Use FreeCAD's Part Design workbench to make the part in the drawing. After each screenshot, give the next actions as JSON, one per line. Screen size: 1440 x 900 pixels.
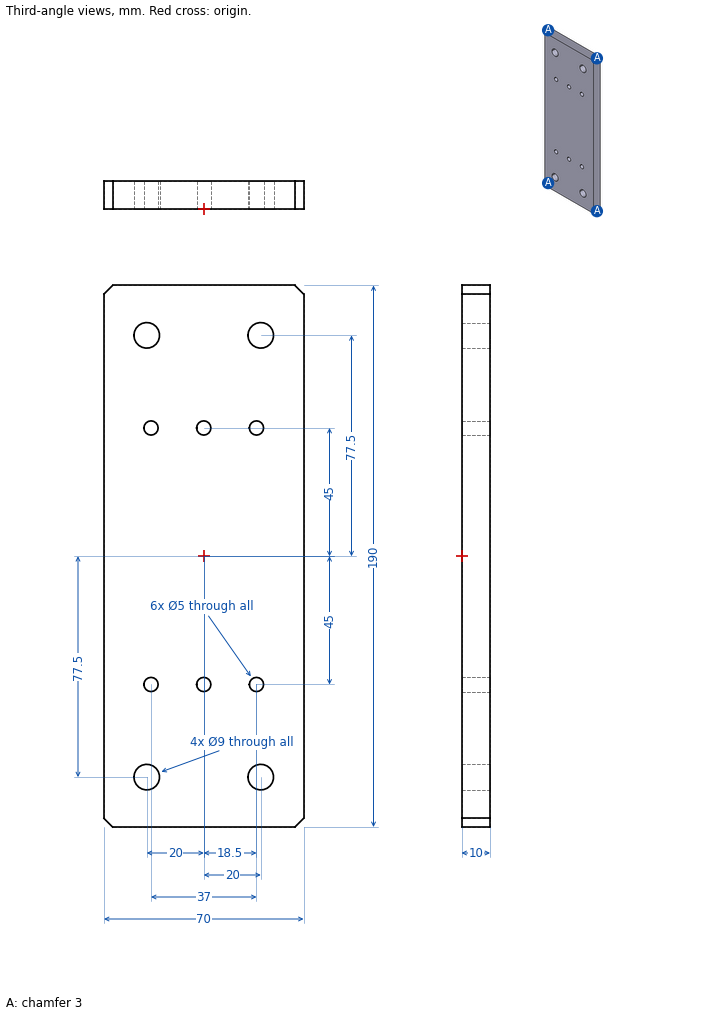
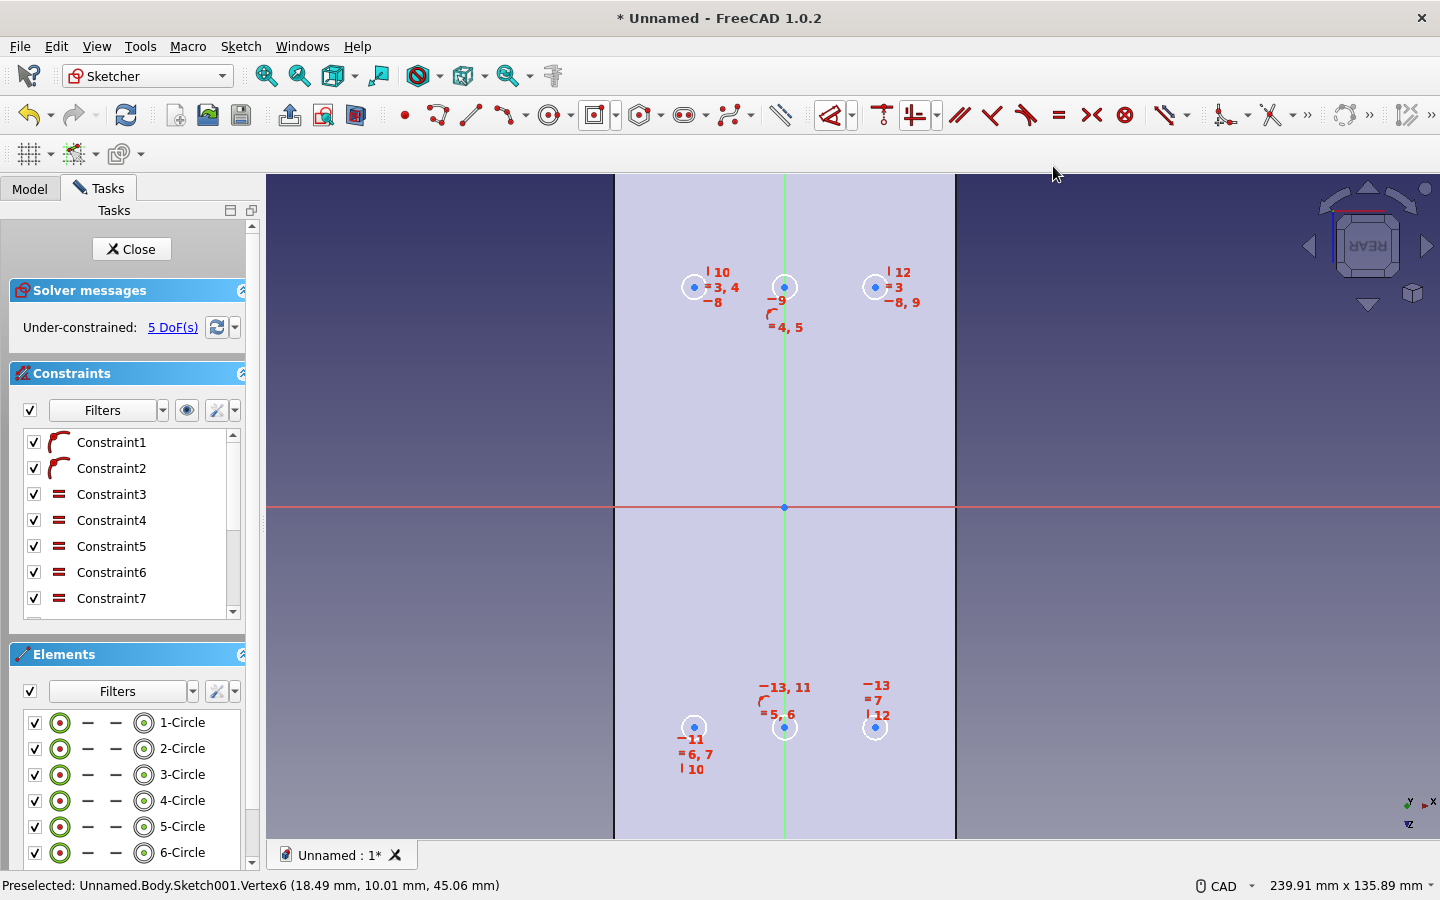
{"action": "scroll", "coordinate": [884, 279], "scroll_direction": "up", "scroll_amount": 3}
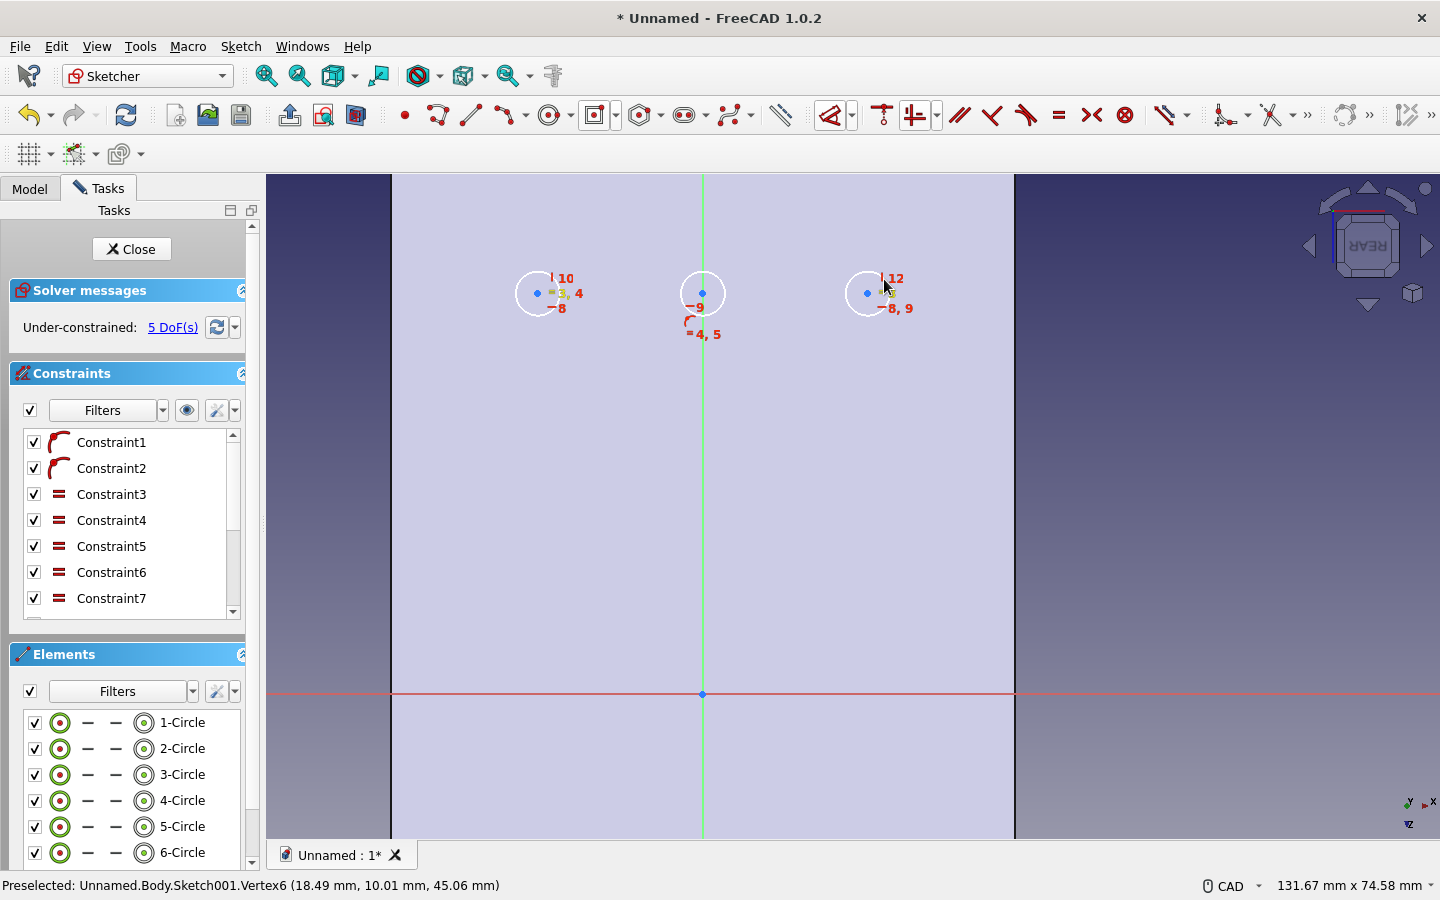
{"action": "left_click", "coordinate": [852, 278]}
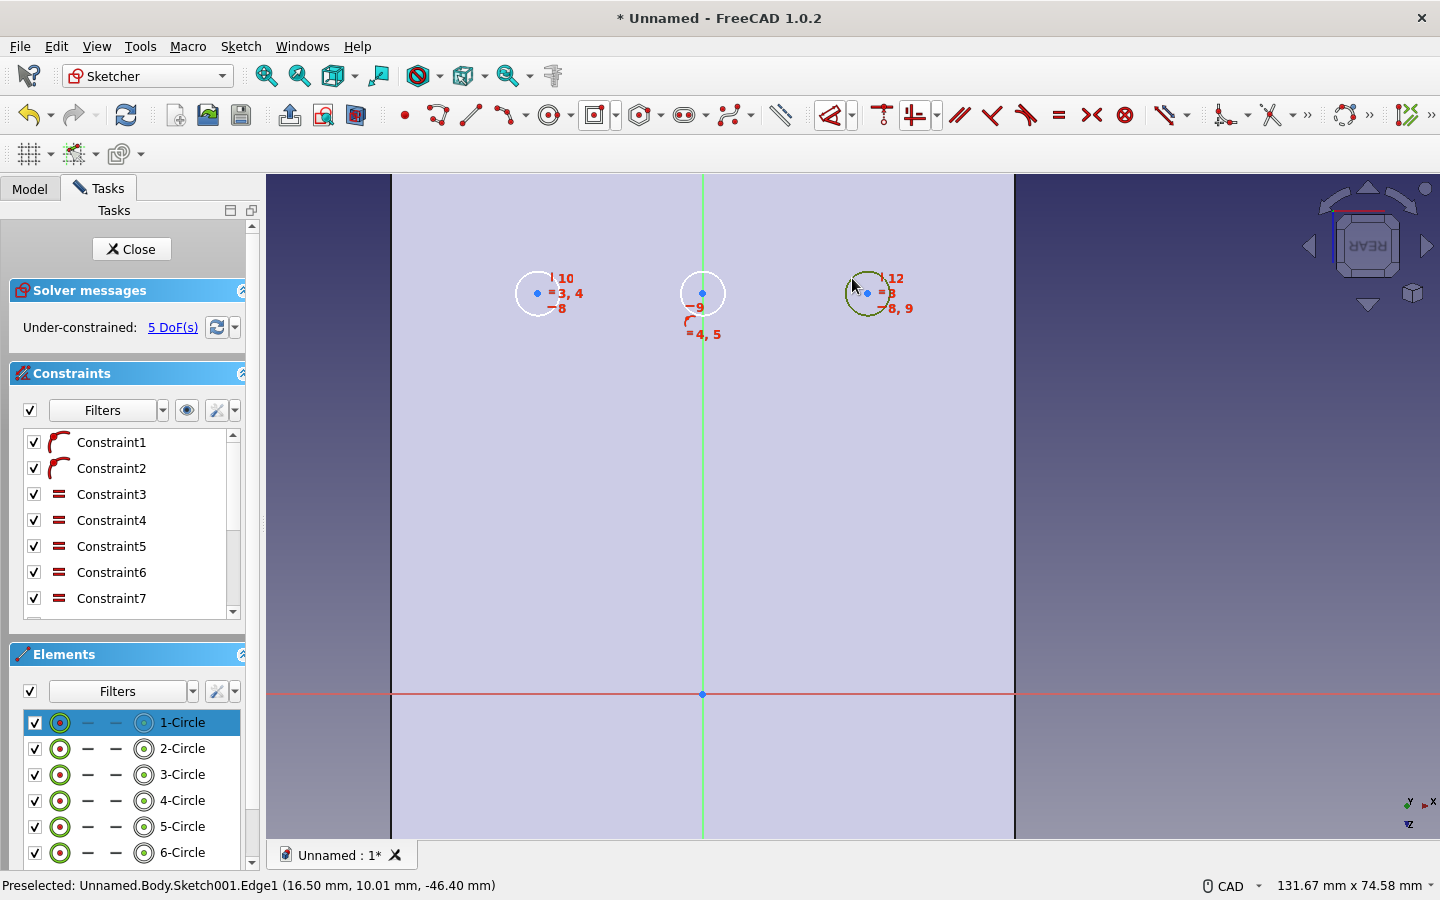
{"action": "key", "text": "k o"}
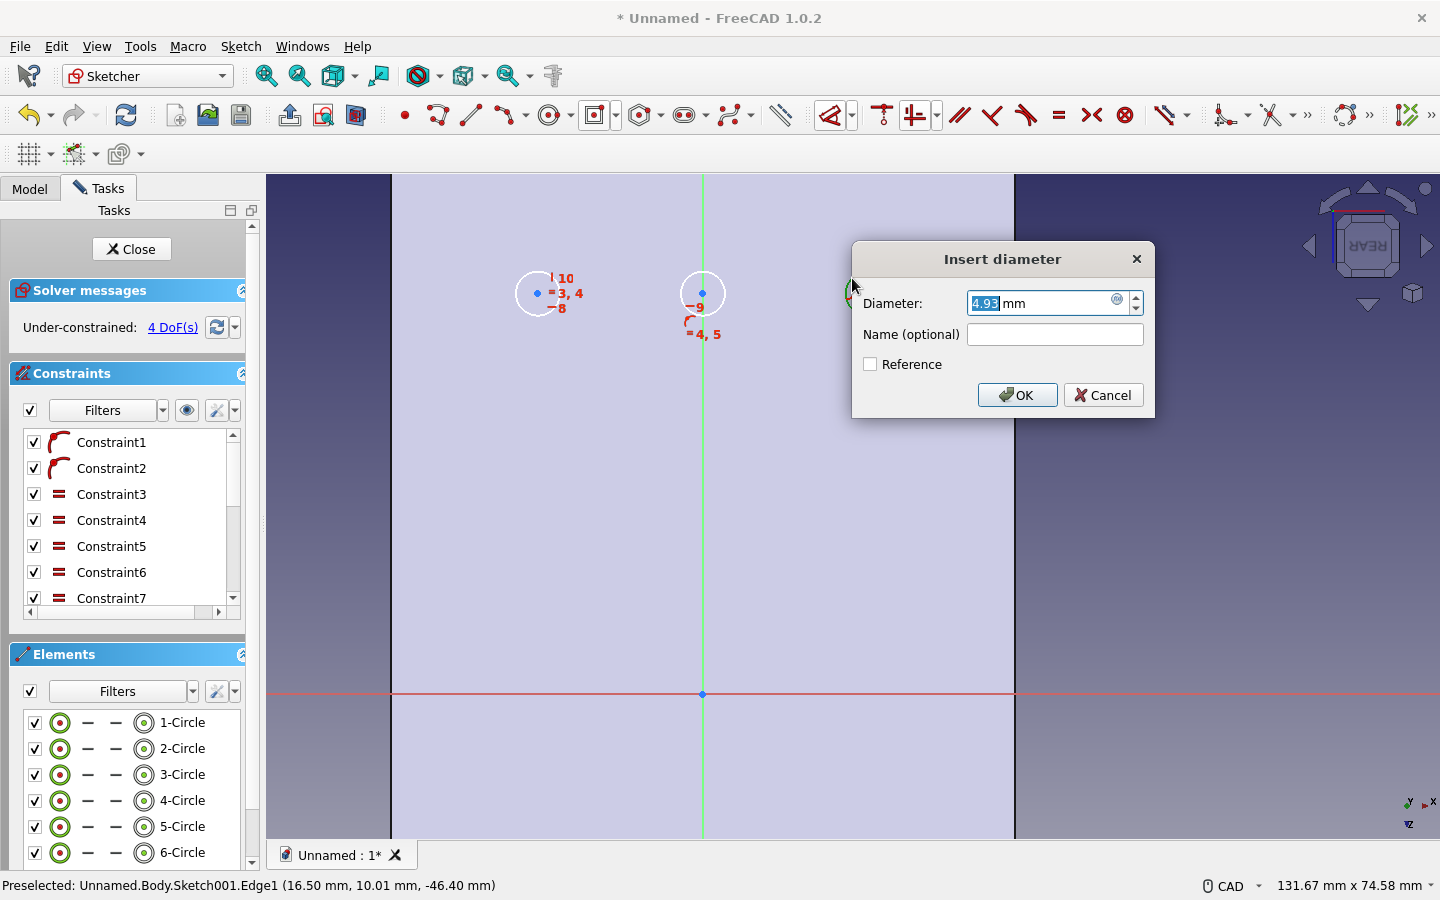
{"action": "type", "text": "5"}
{"action": "key", "text": "Return"}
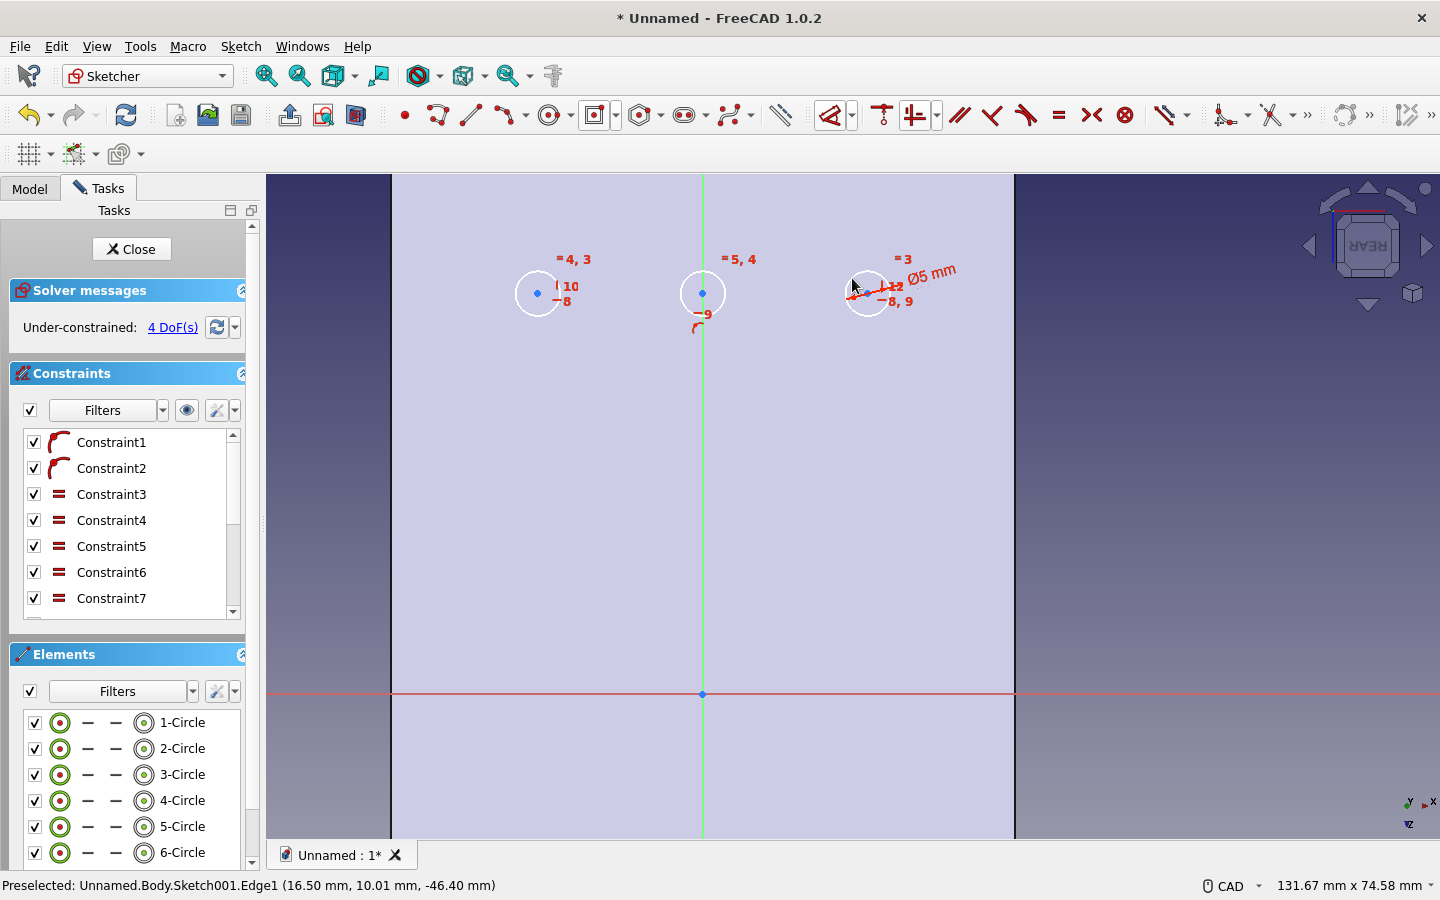
{"action": "left_click", "coordinate": [868, 294]}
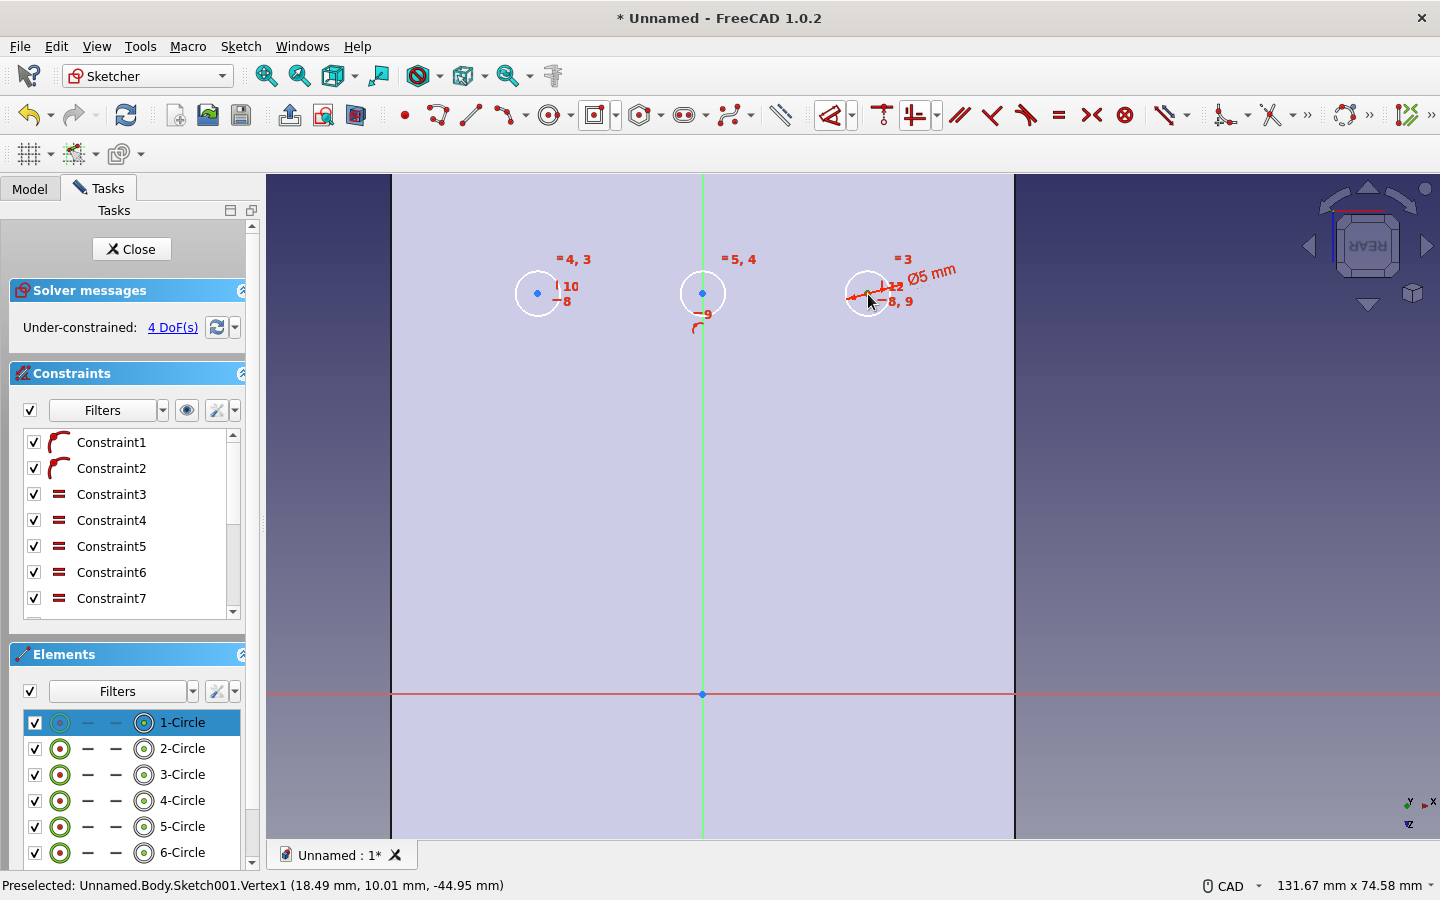
{"action": "key", "text": "i"}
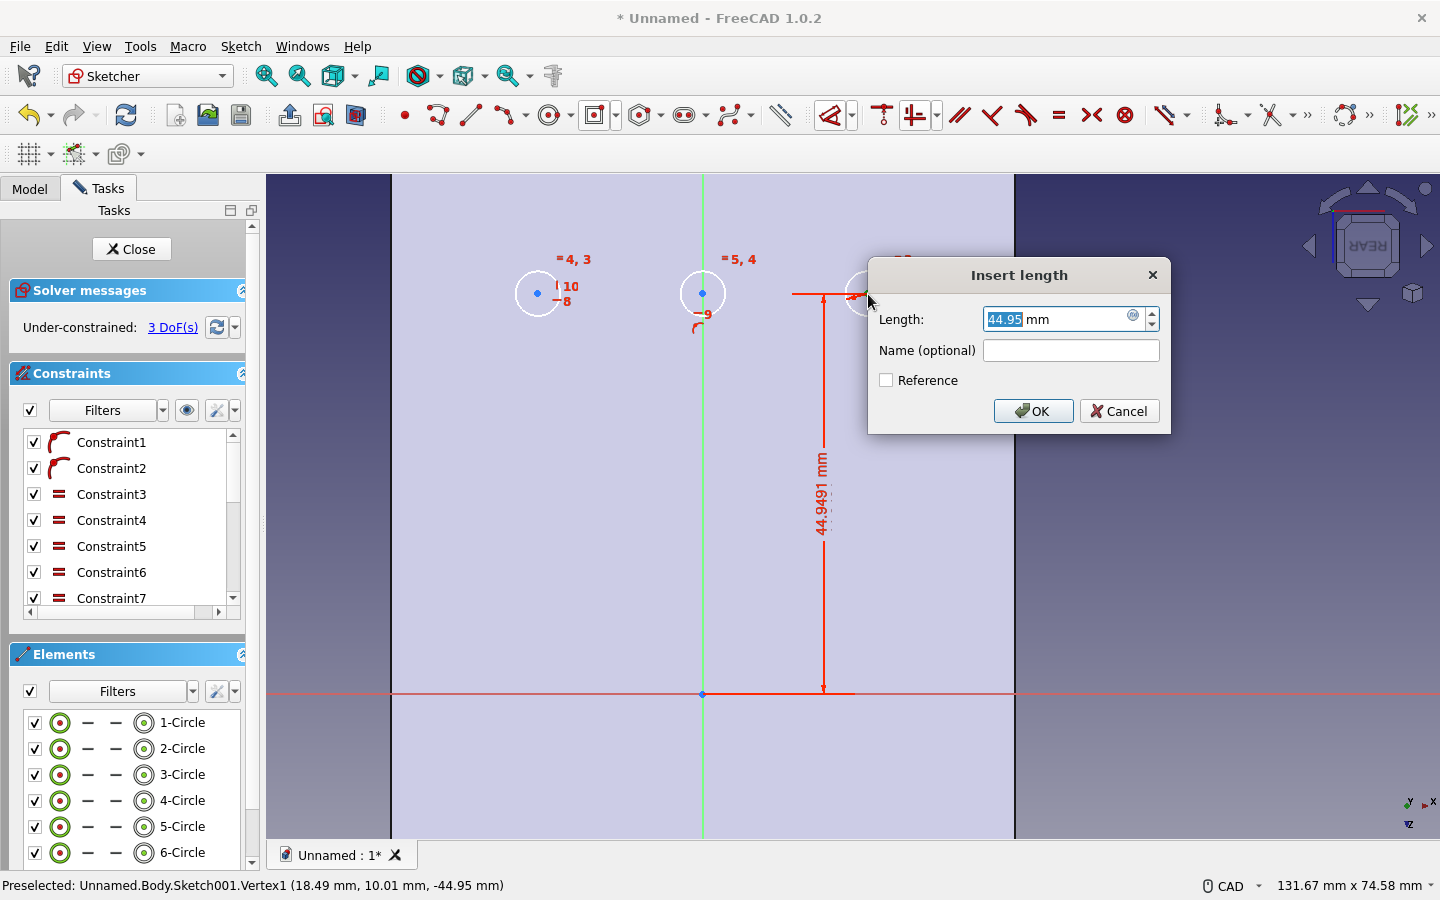
{"action": "type", "text": "45"}
{"action": "key", "text": "Return"}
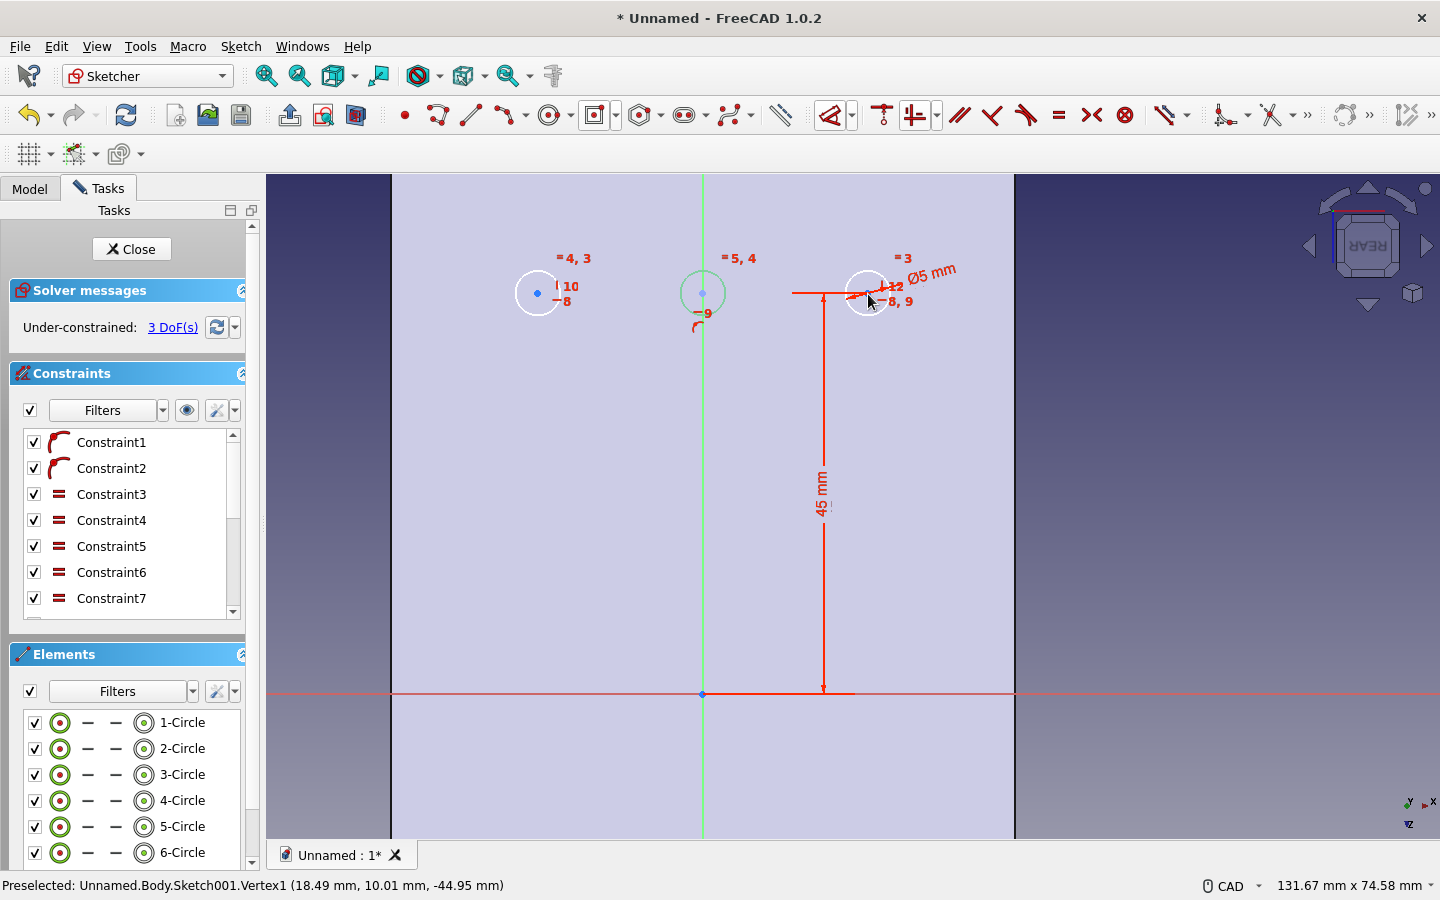
{"action": "scroll", "coordinate": [884, 278], "scroll_direction": "down", "scroll_amount": 3}